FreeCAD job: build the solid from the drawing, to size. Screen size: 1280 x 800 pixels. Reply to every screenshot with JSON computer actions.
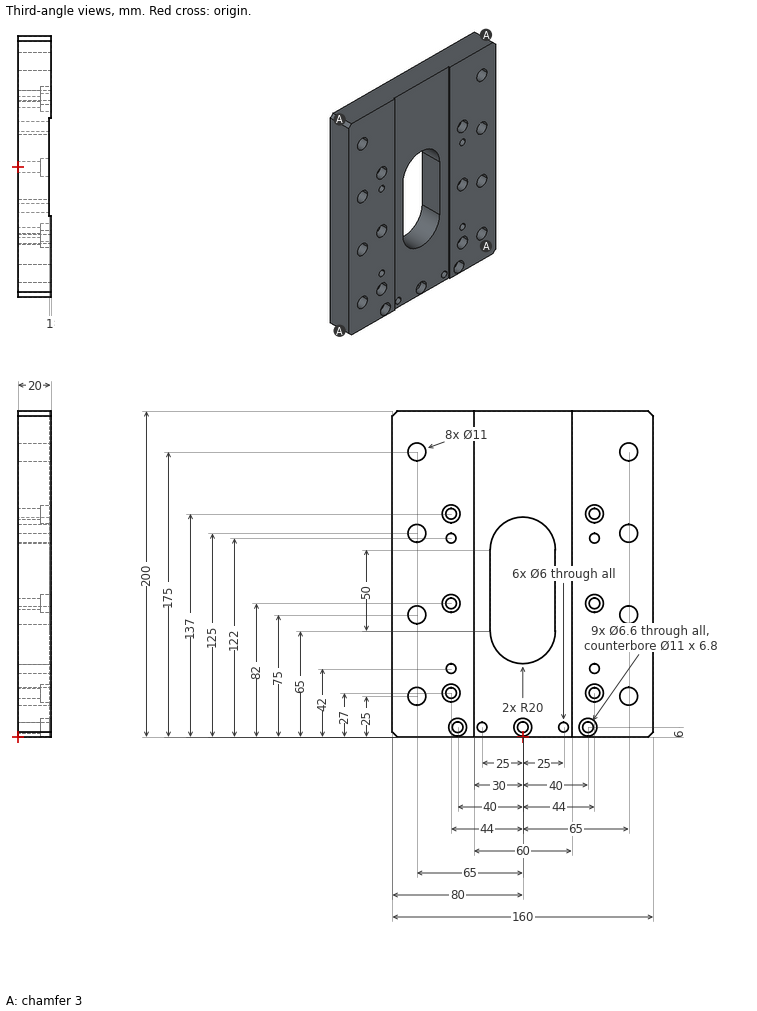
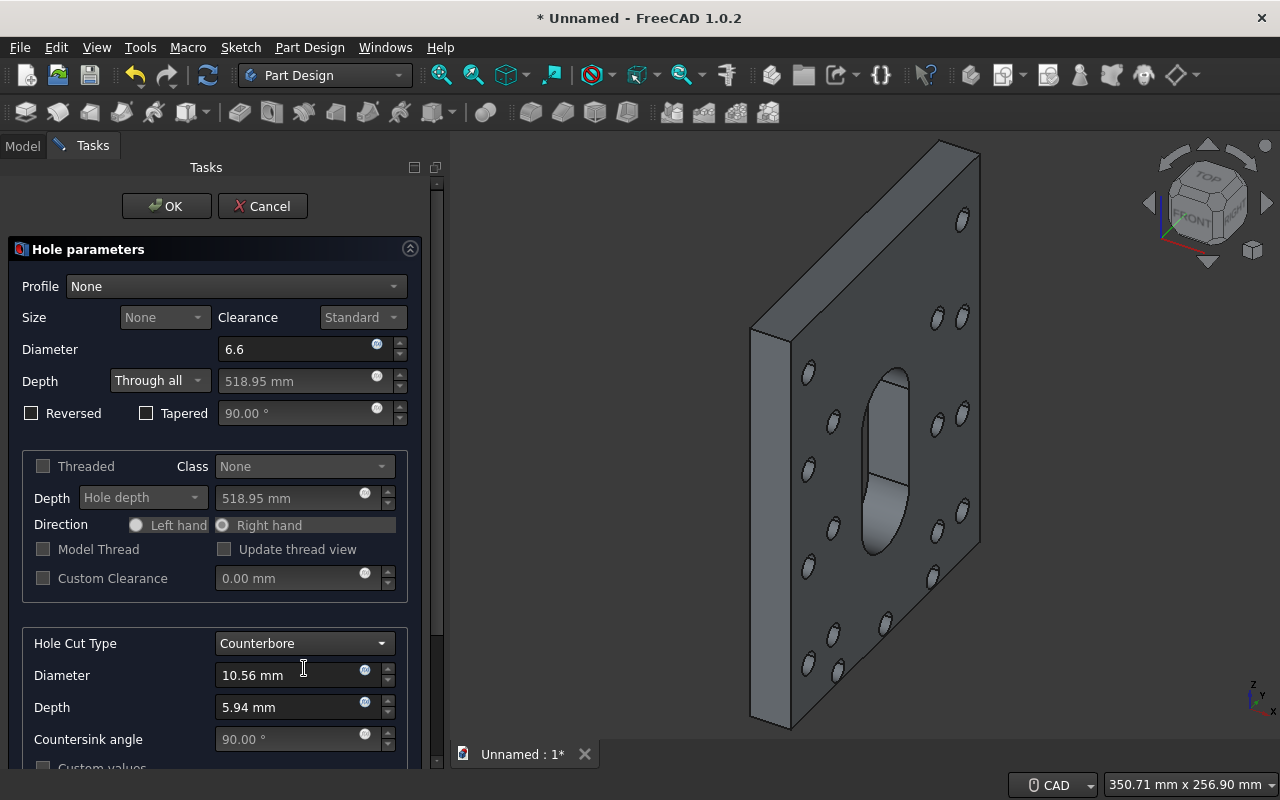
{"action": "triple_click", "coordinate": [298, 675]}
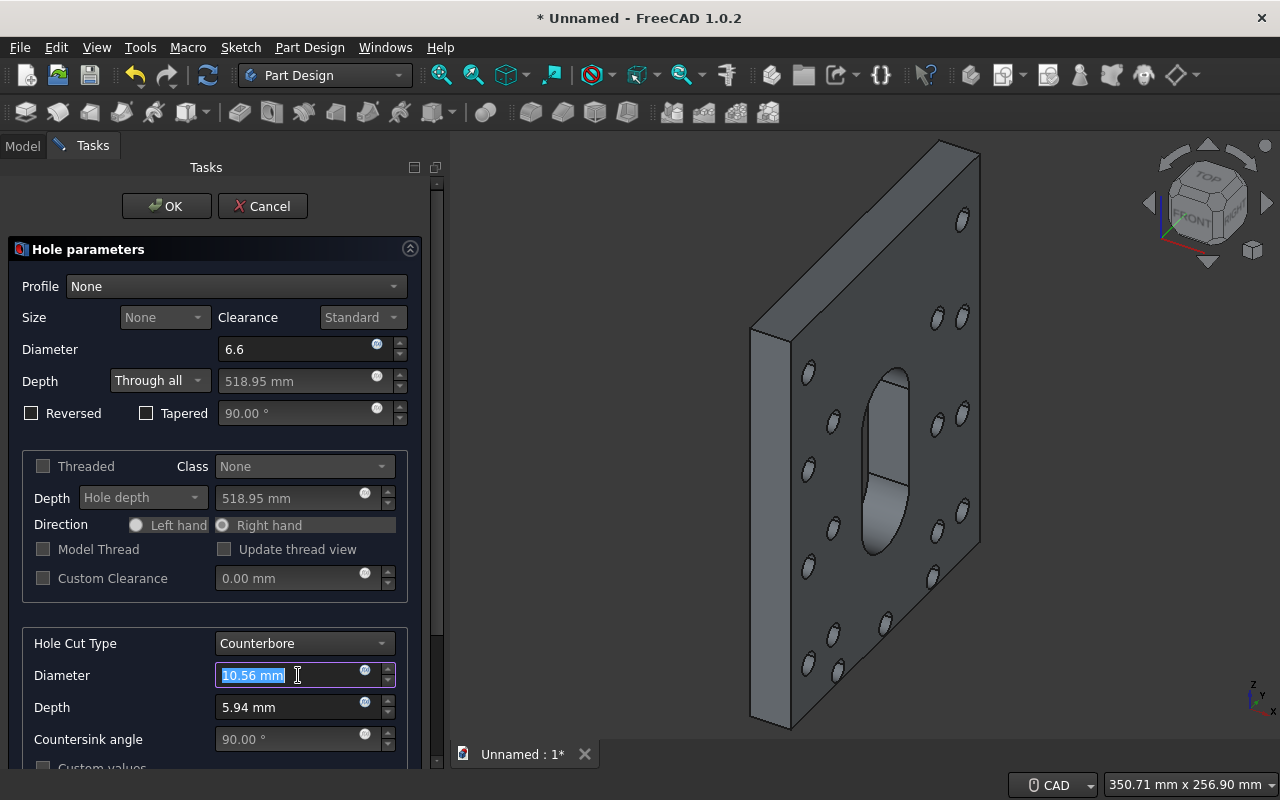
{"action": "type", "text": "11"}
{"action": "key", "text": "Tab"}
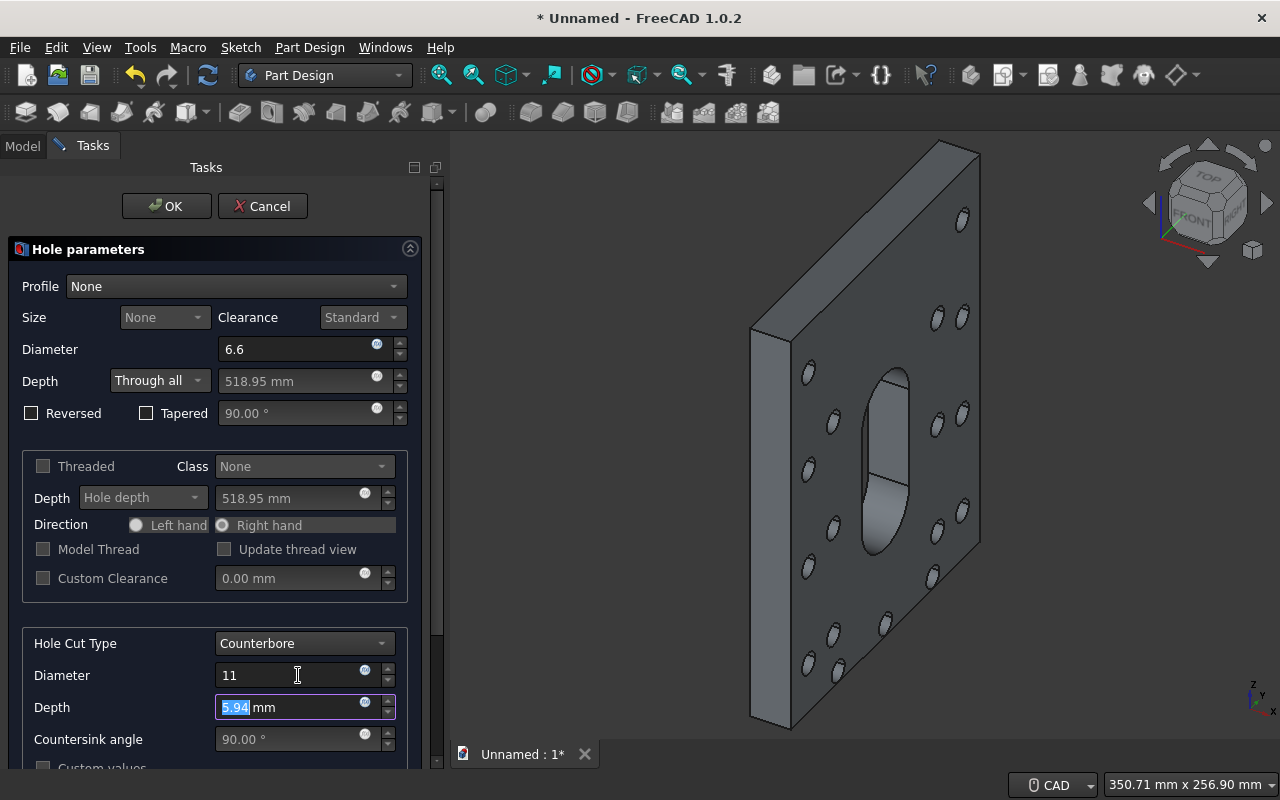
{"action": "type", "text": "6.8"}
{"action": "key", "text": "Tab"}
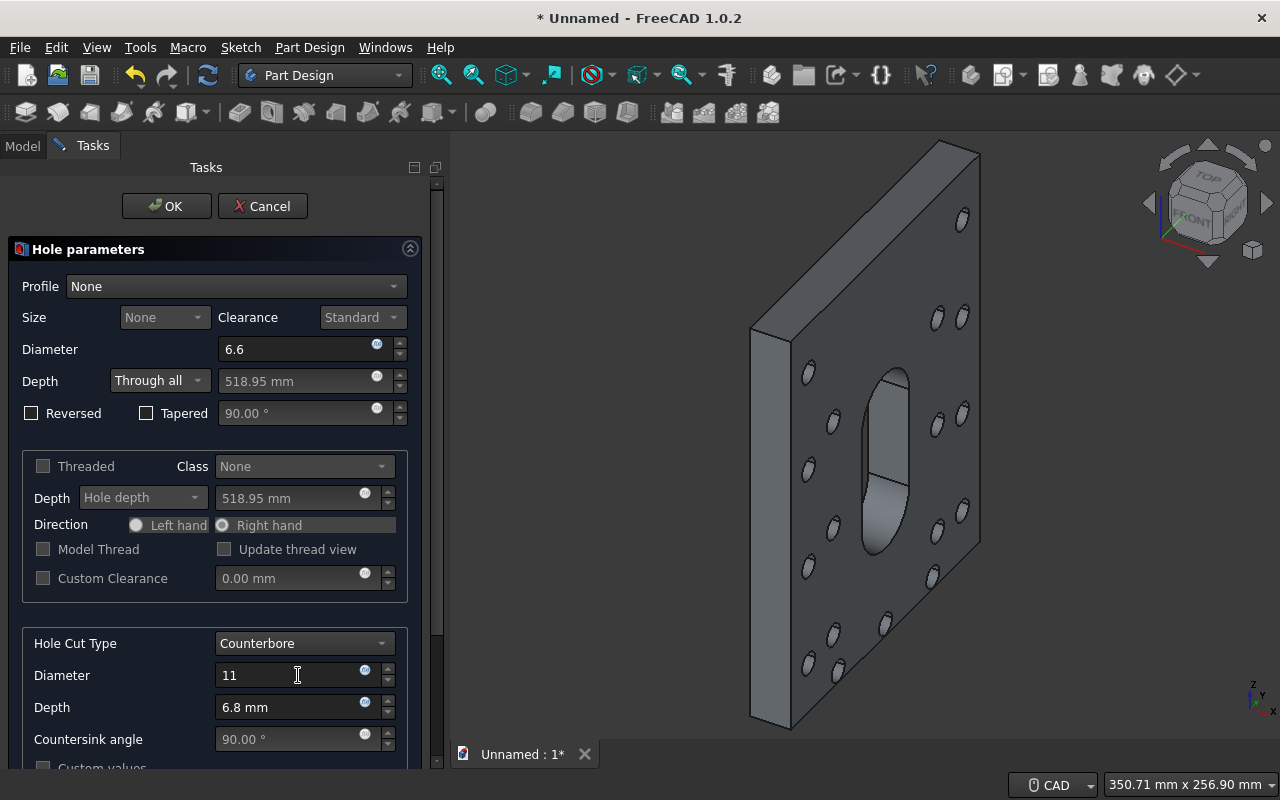
{"action": "left_click", "coordinate": [167, 206]}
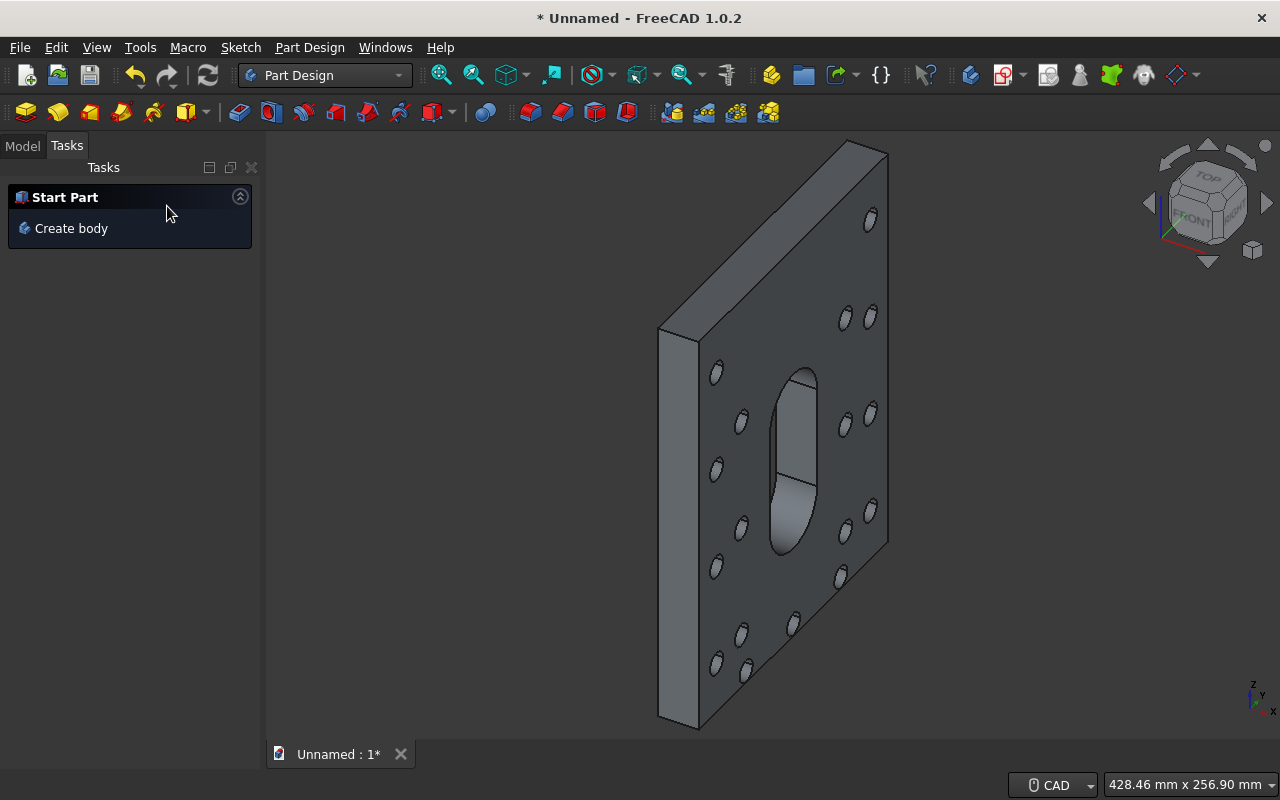
{"action": "left_click", "coordinate": [766, 357]}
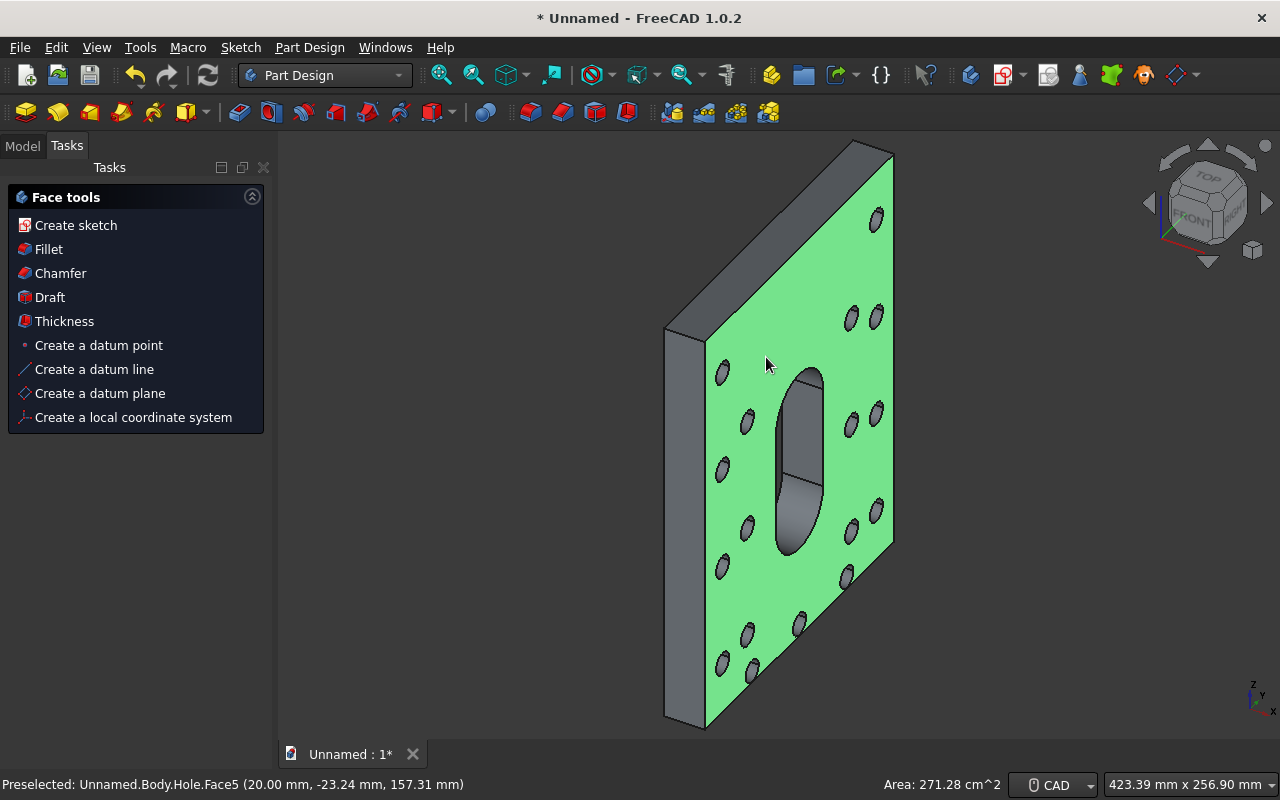
{"action": "left_click", "coordinate": [1004, 76]}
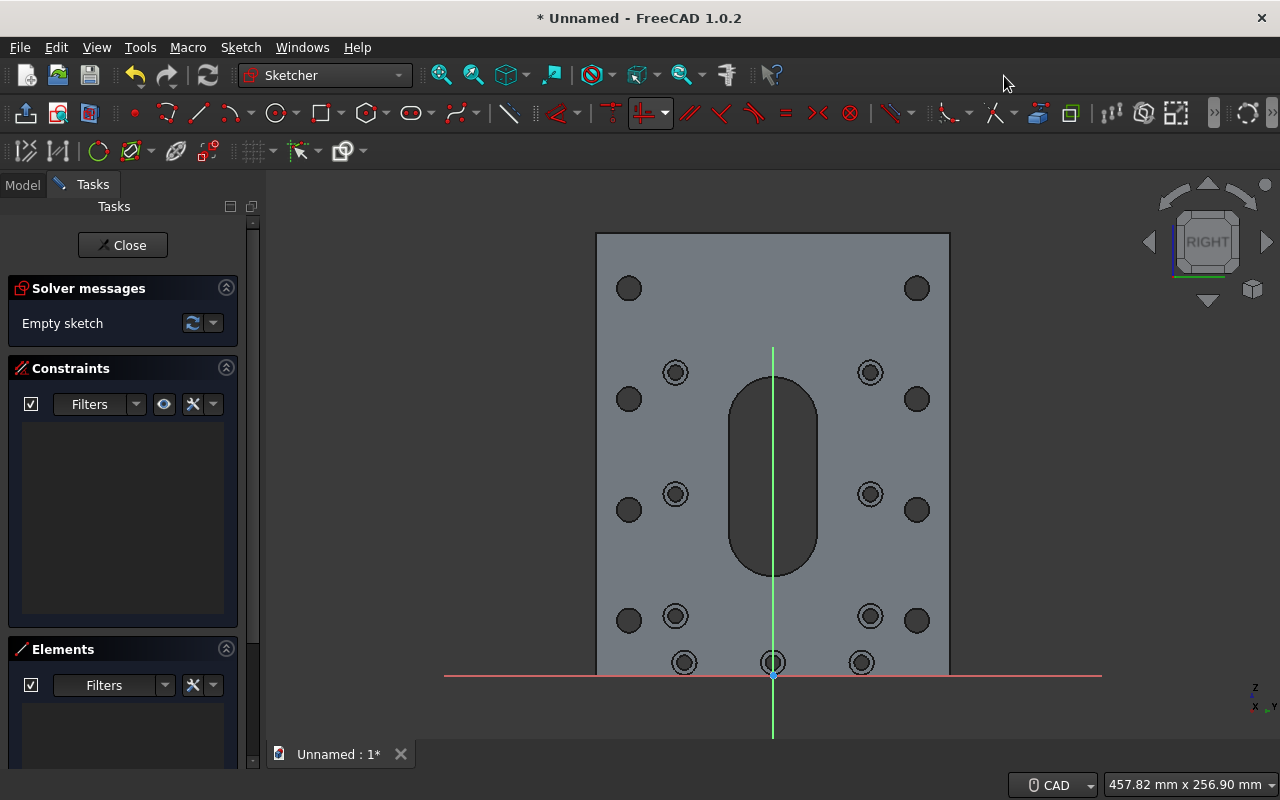
{"action": "key", "text": "g c"}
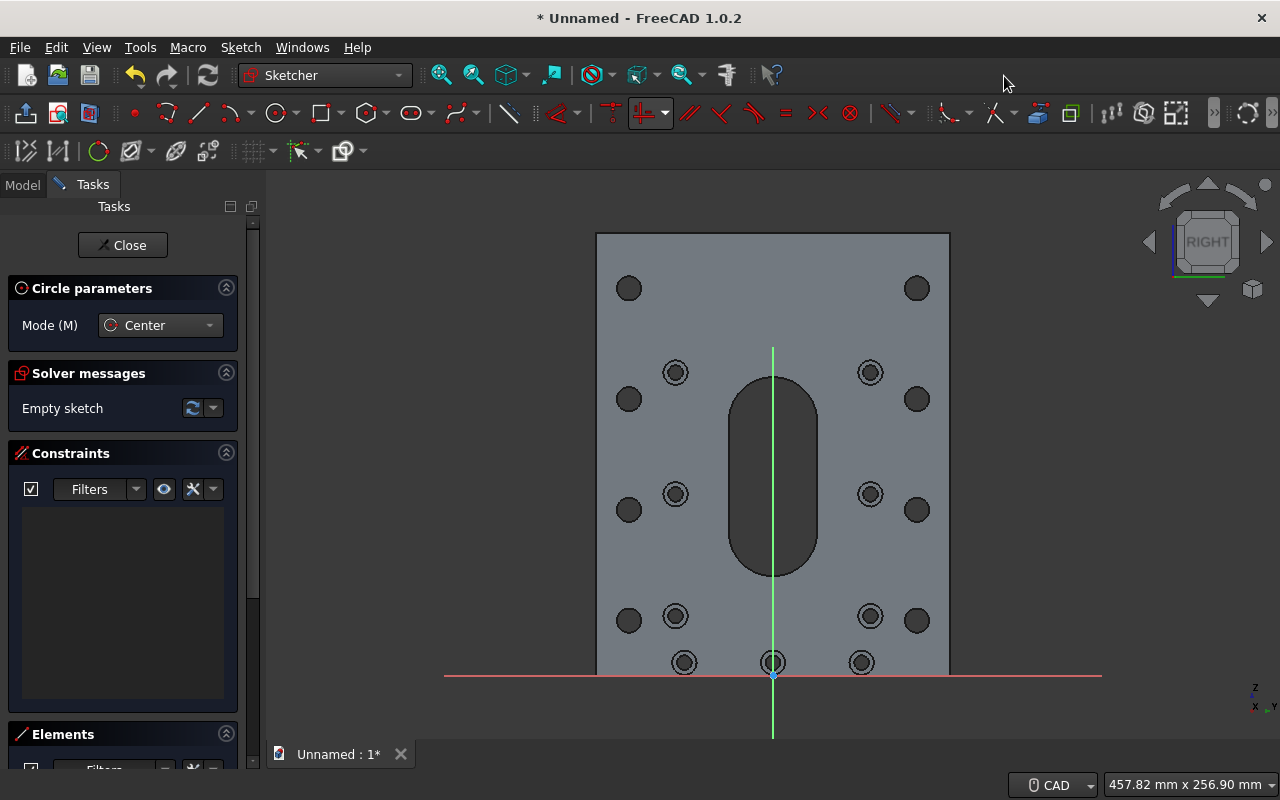
{"action": "scroll", "coordinate": [828, 663], "scroll_direction": "up", "scroll_amount": 7}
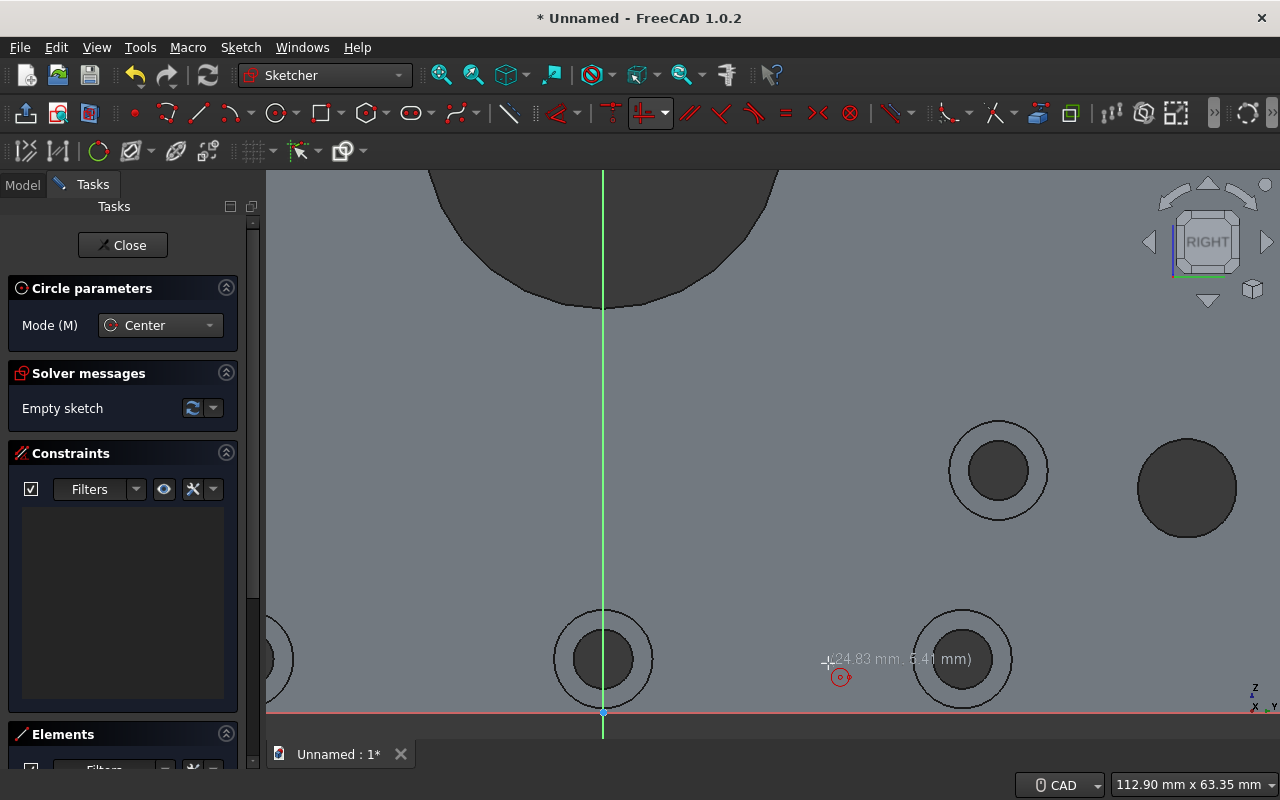
{"action": "scroll", "coordinate": [748, 585], "scroll_direction": "down", "scroll_amount": 6}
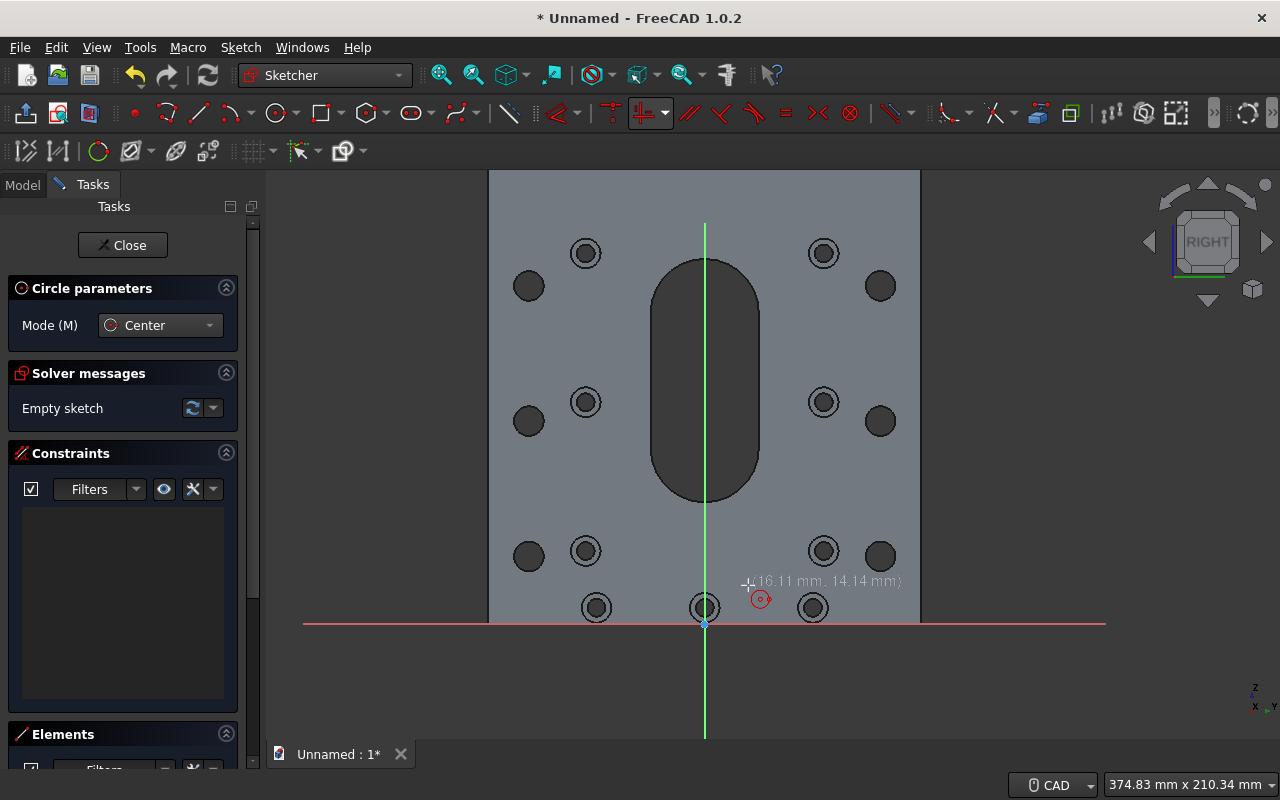
{"action": "left_click", "coordinate": [772, 608]}
{"action": "mouse_move", "coordinate": [778, 602]}